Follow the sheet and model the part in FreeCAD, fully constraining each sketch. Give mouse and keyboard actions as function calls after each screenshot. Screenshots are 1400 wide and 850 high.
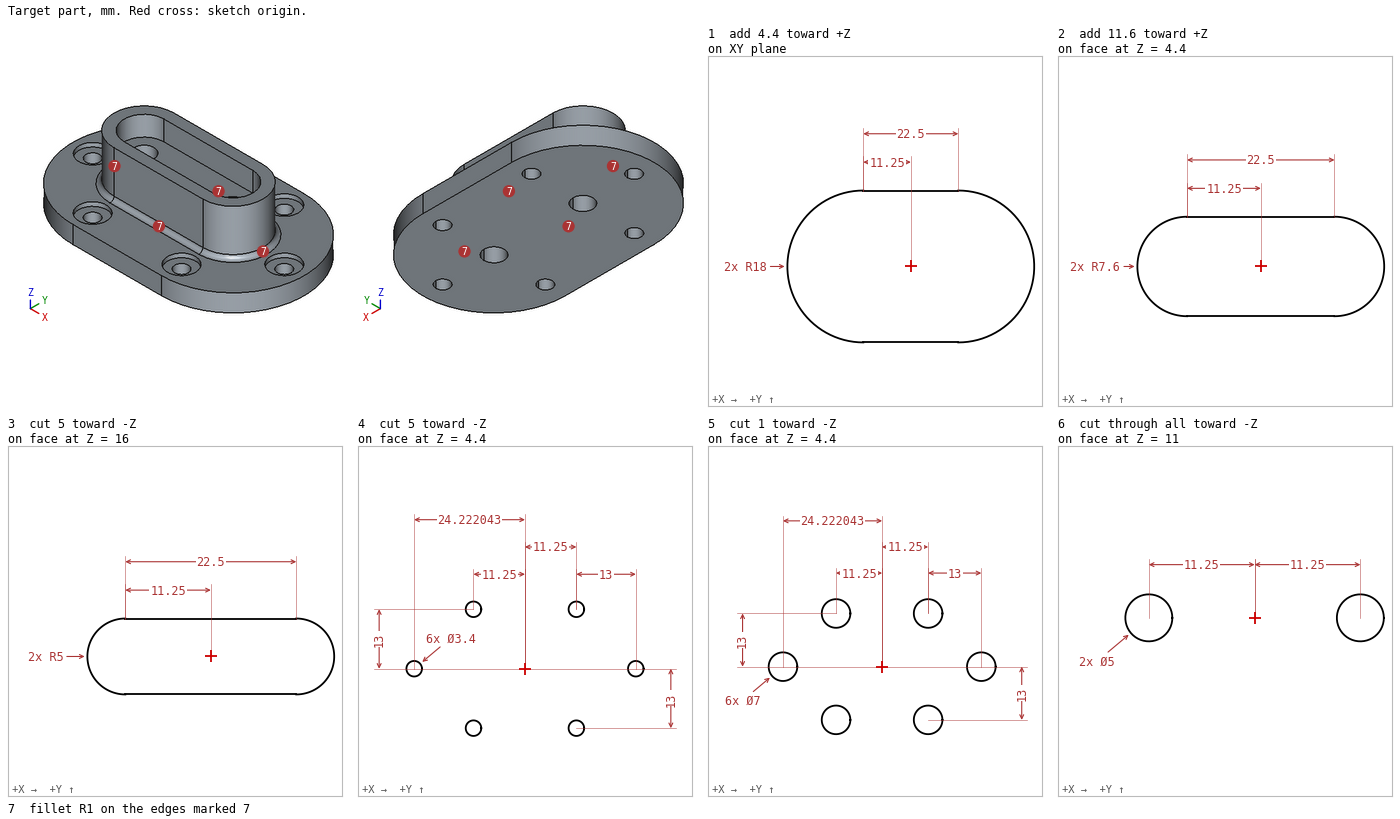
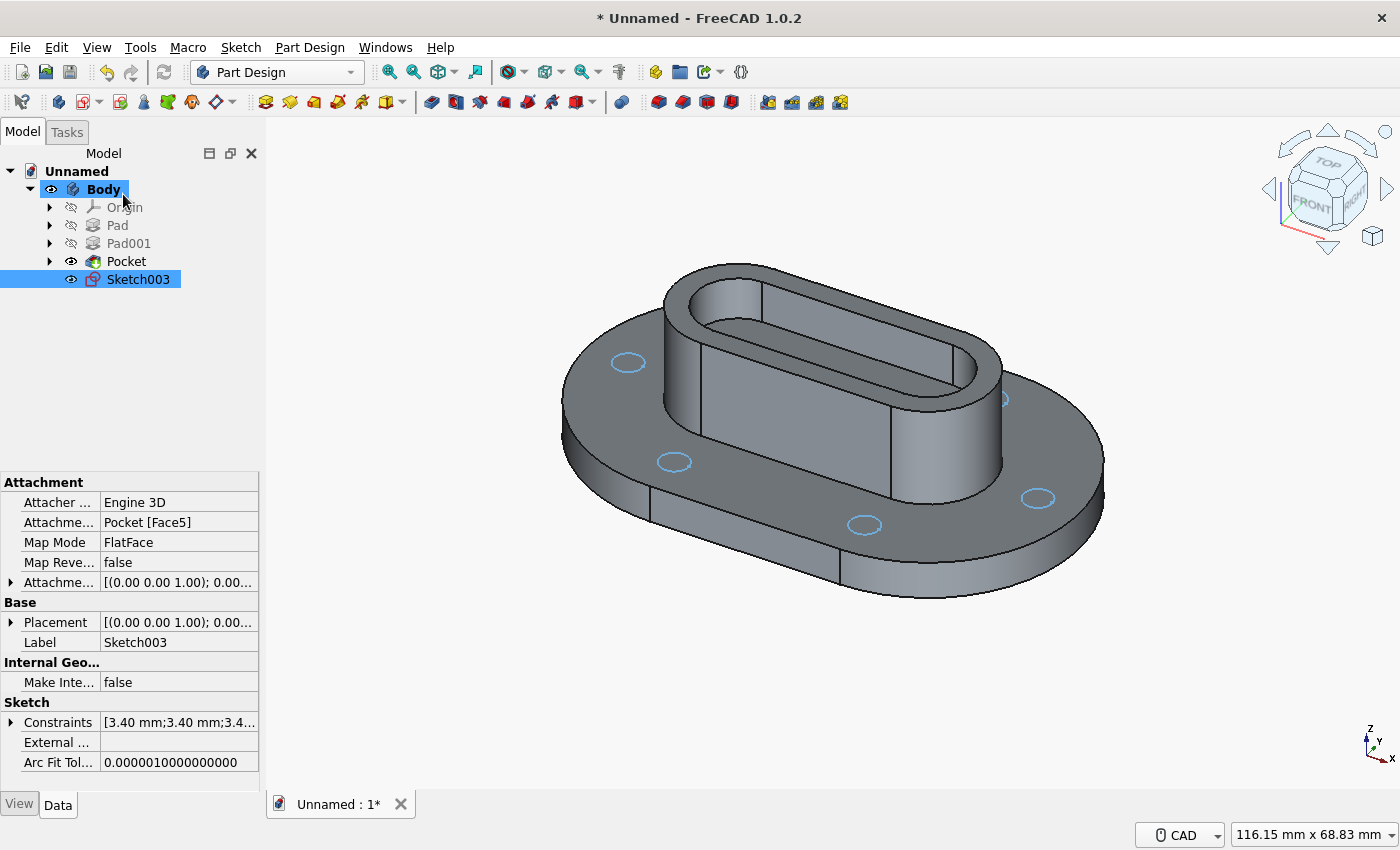
click(432, 102)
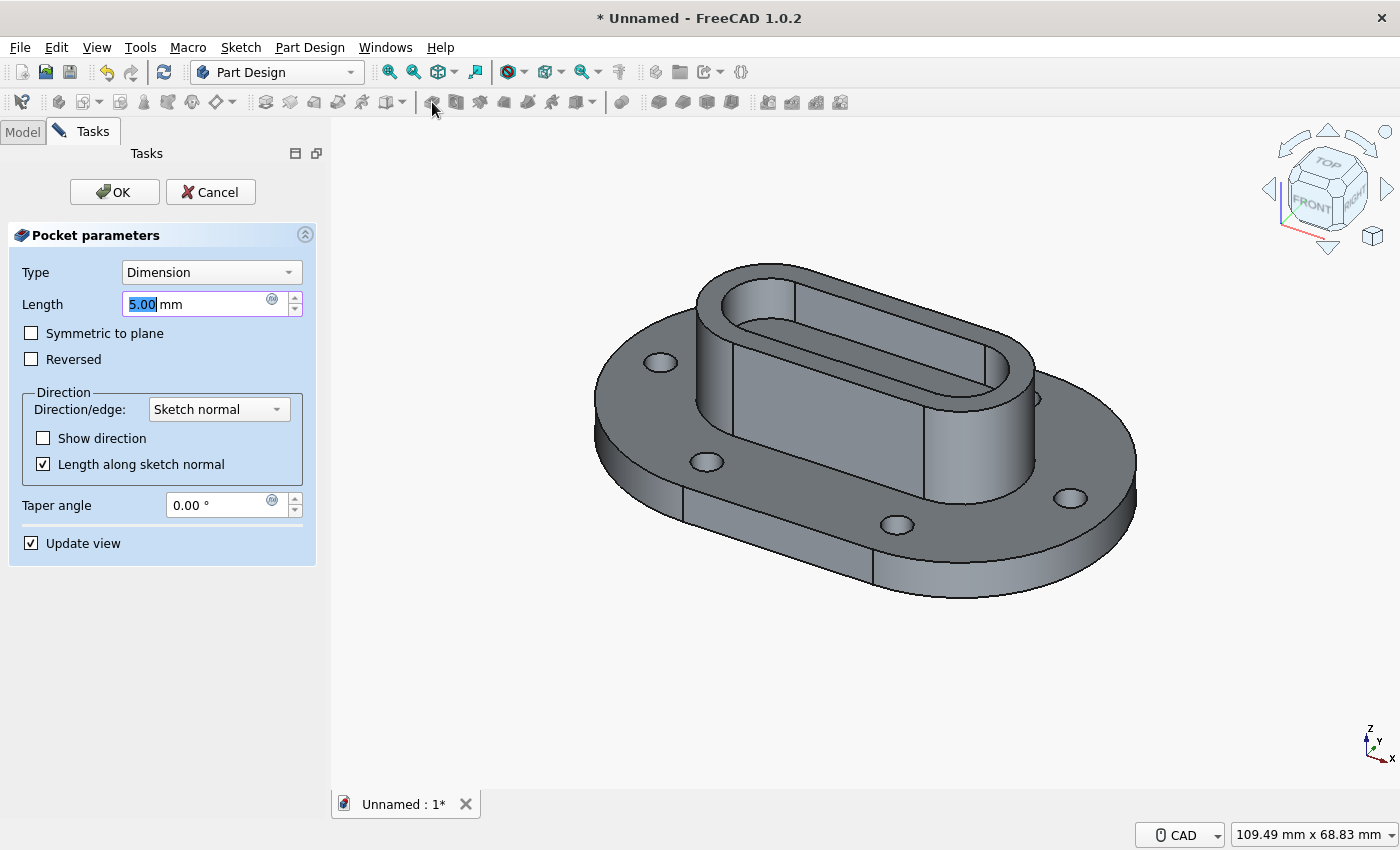
text(5)
key(Tab)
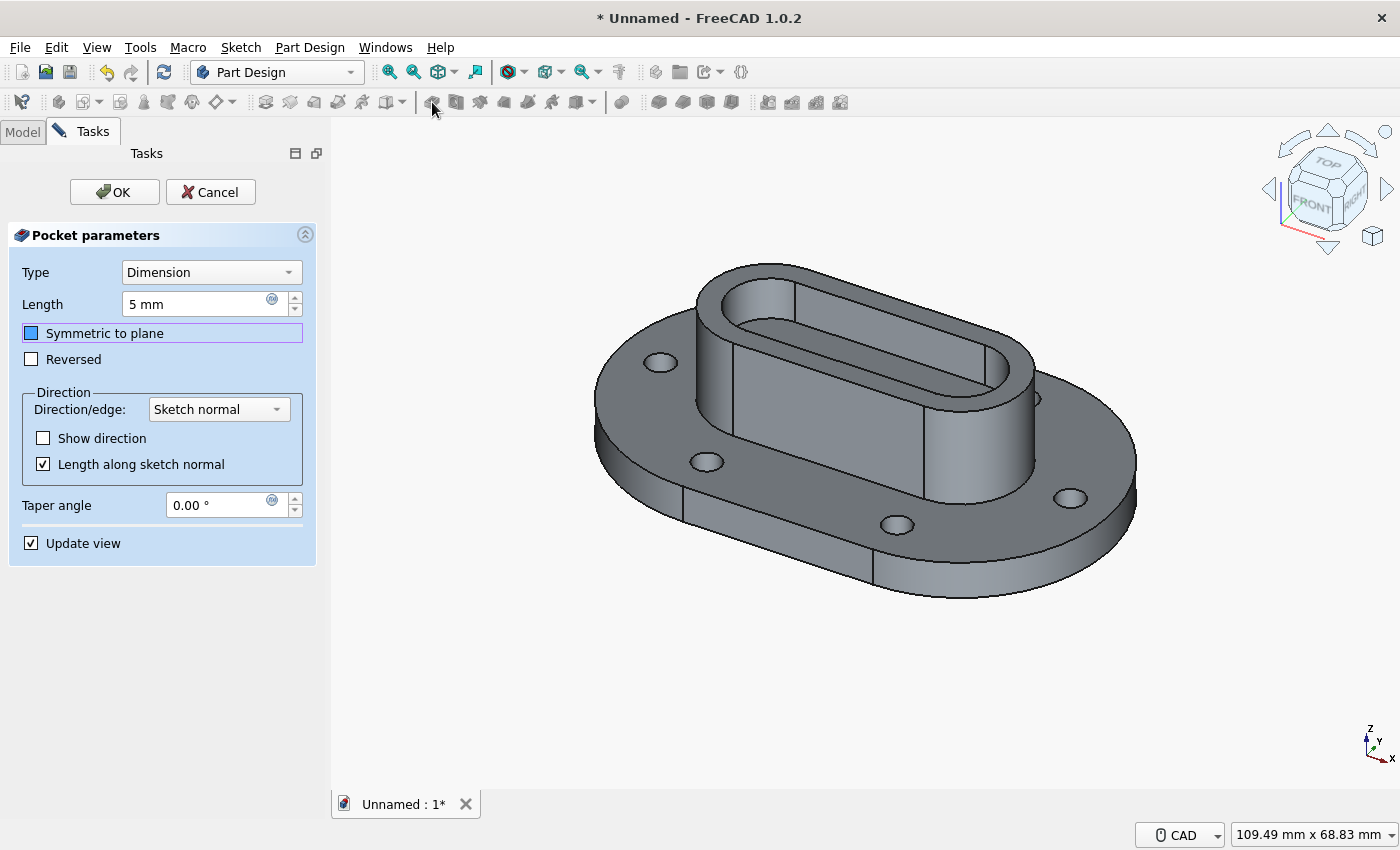
click(115, 192)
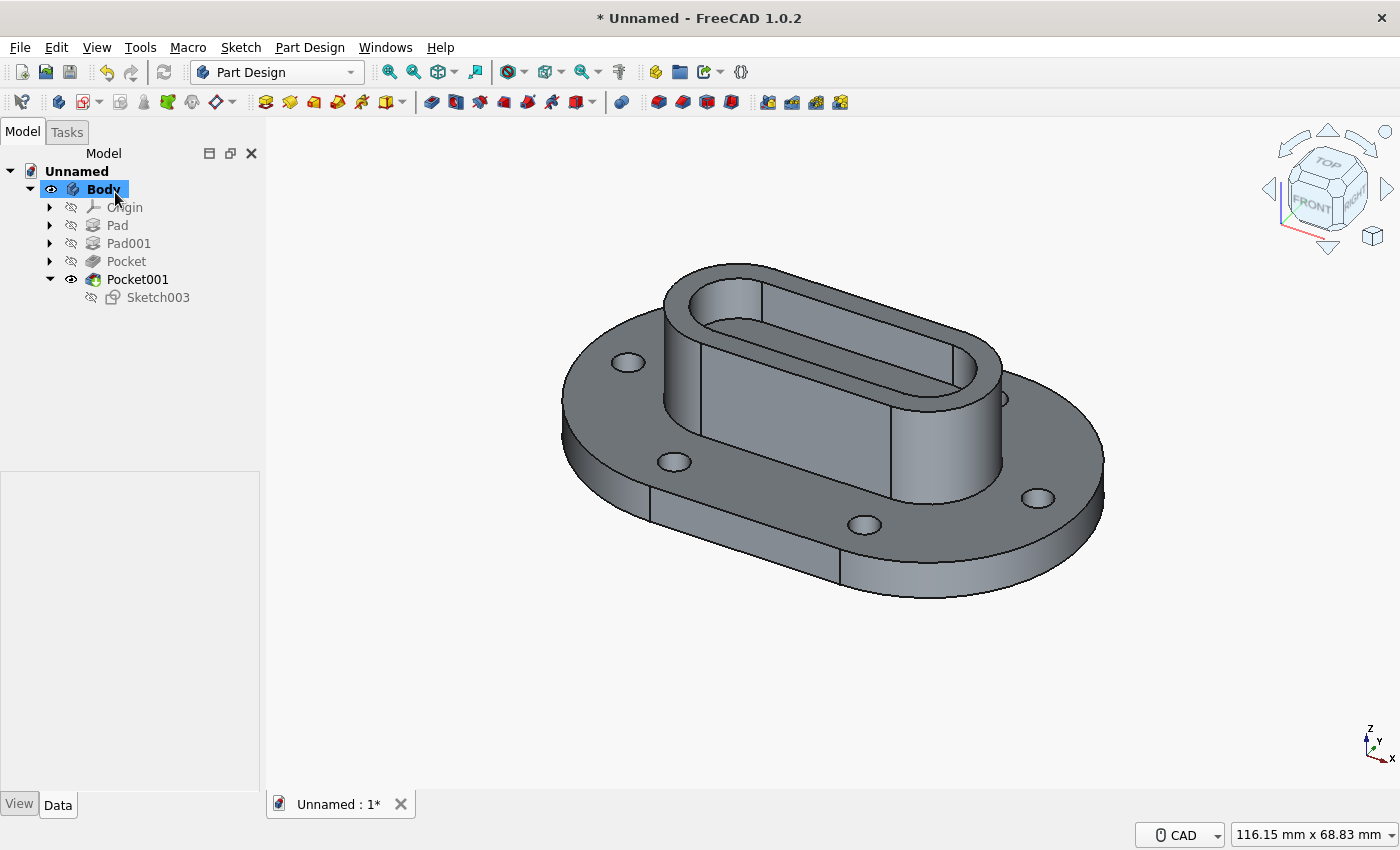
click(641, 433)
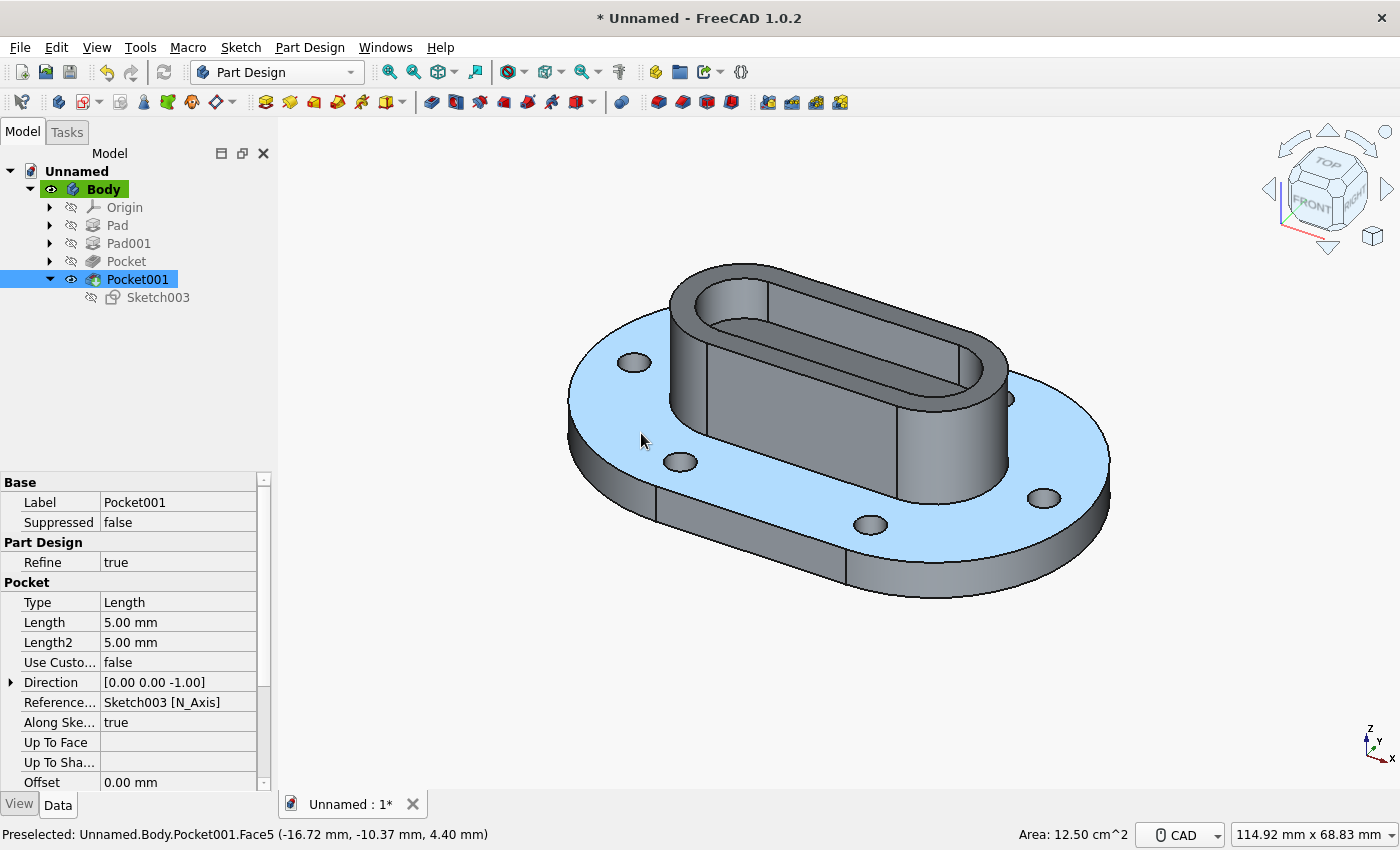
click(84, 102)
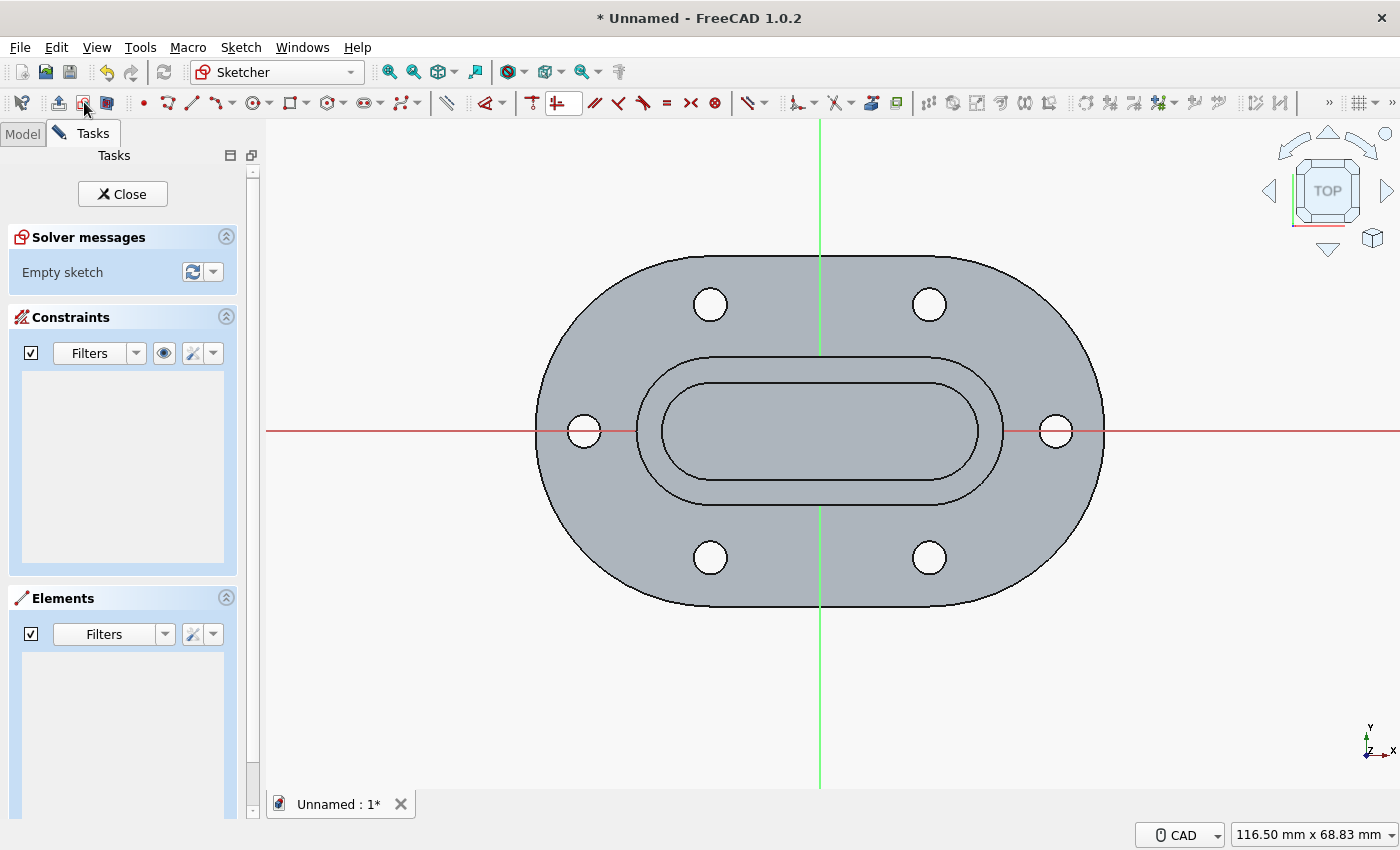
click(108, 104)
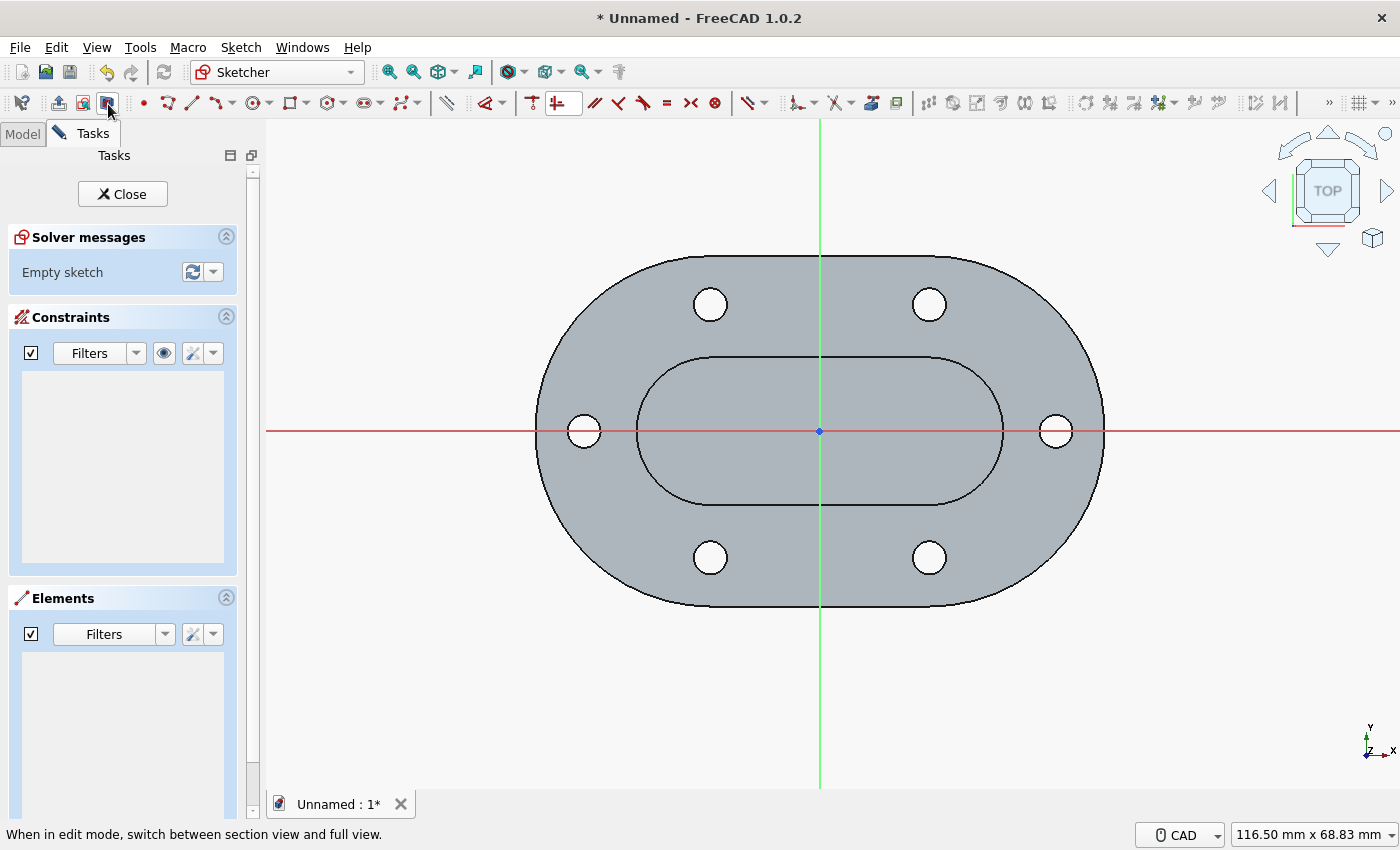
click(254, 104)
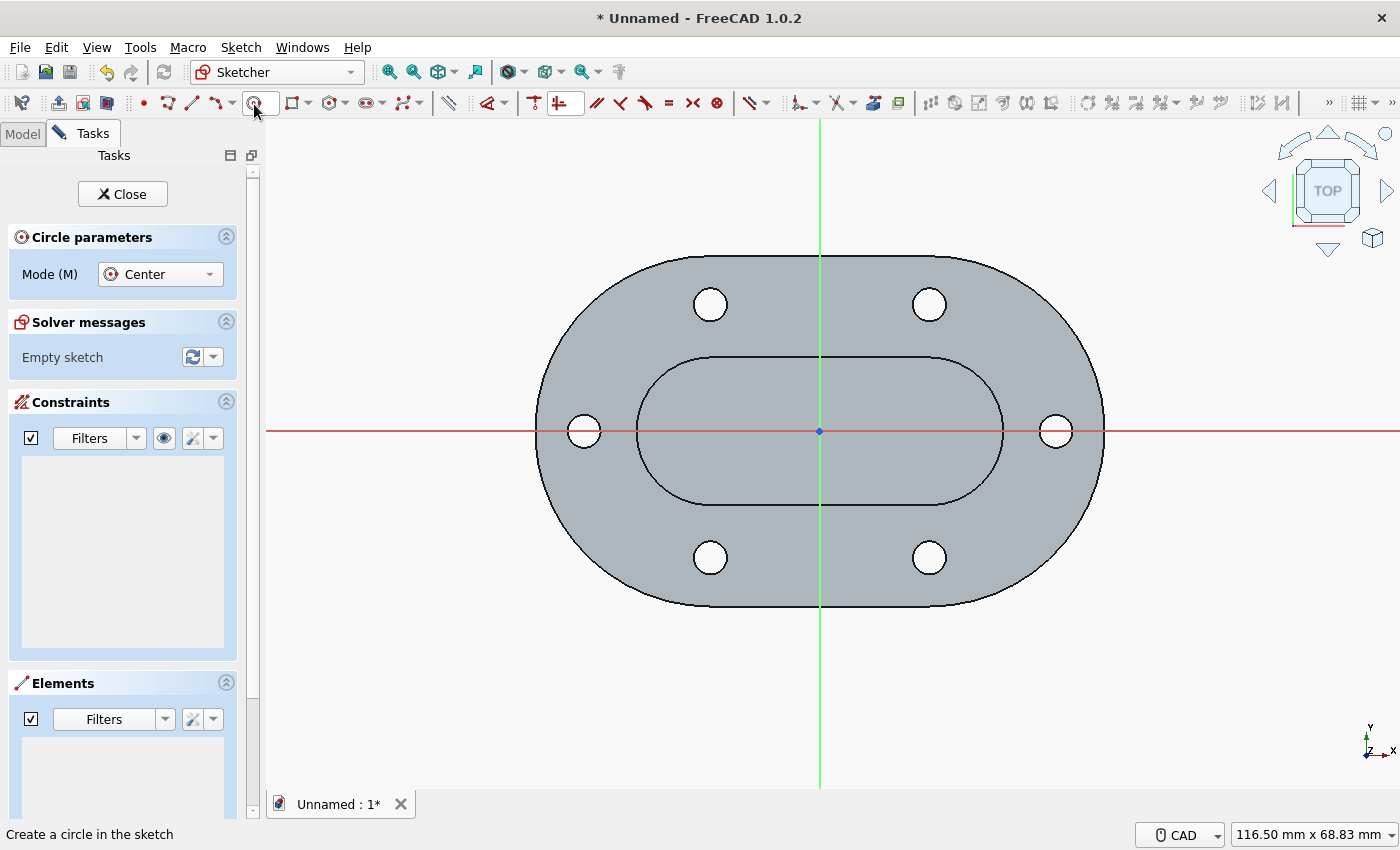
click(584, 431)
move(608, 407)